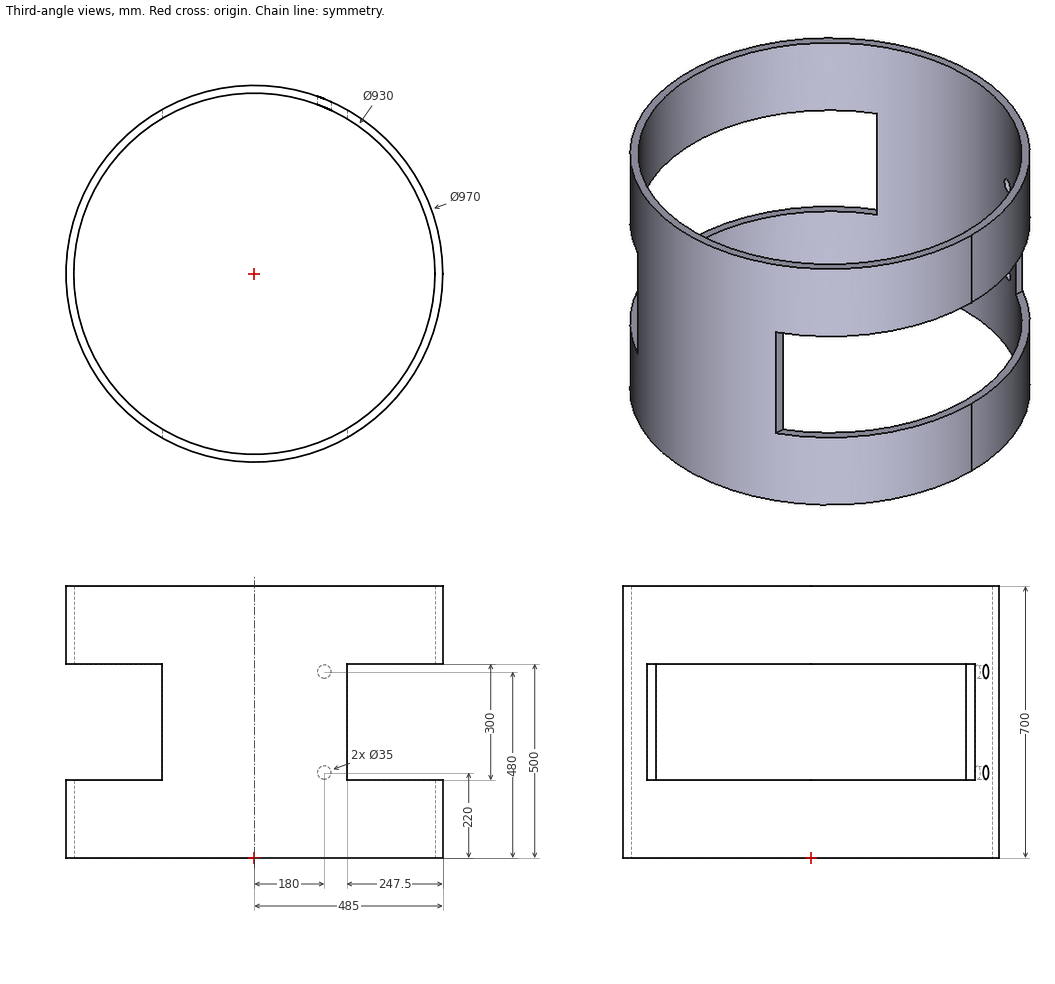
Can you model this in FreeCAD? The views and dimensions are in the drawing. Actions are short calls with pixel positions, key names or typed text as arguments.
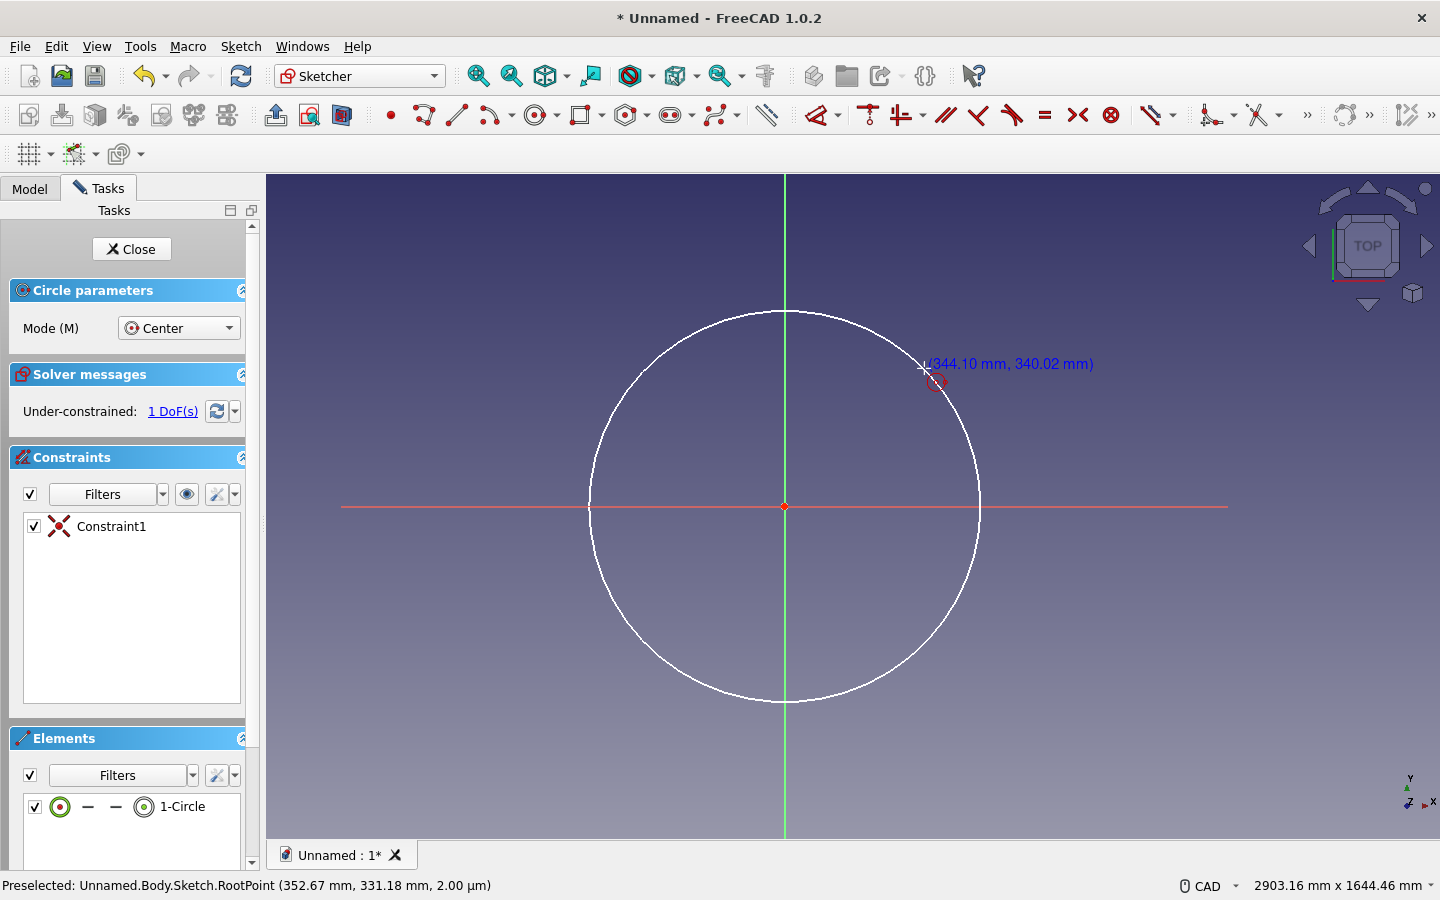
click(785, 506)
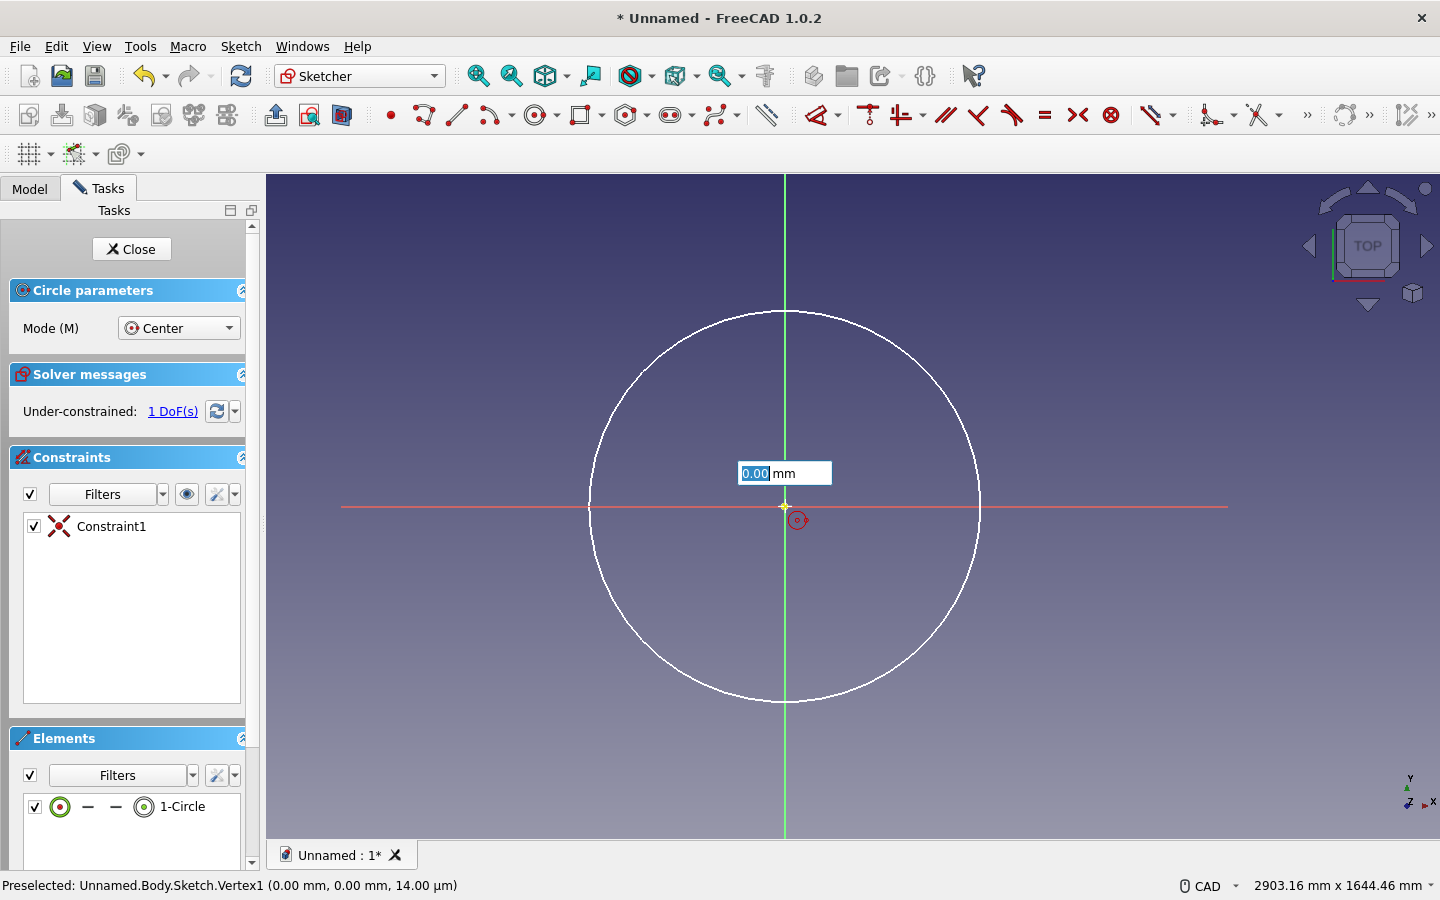
scroll(918, 374, up, 4)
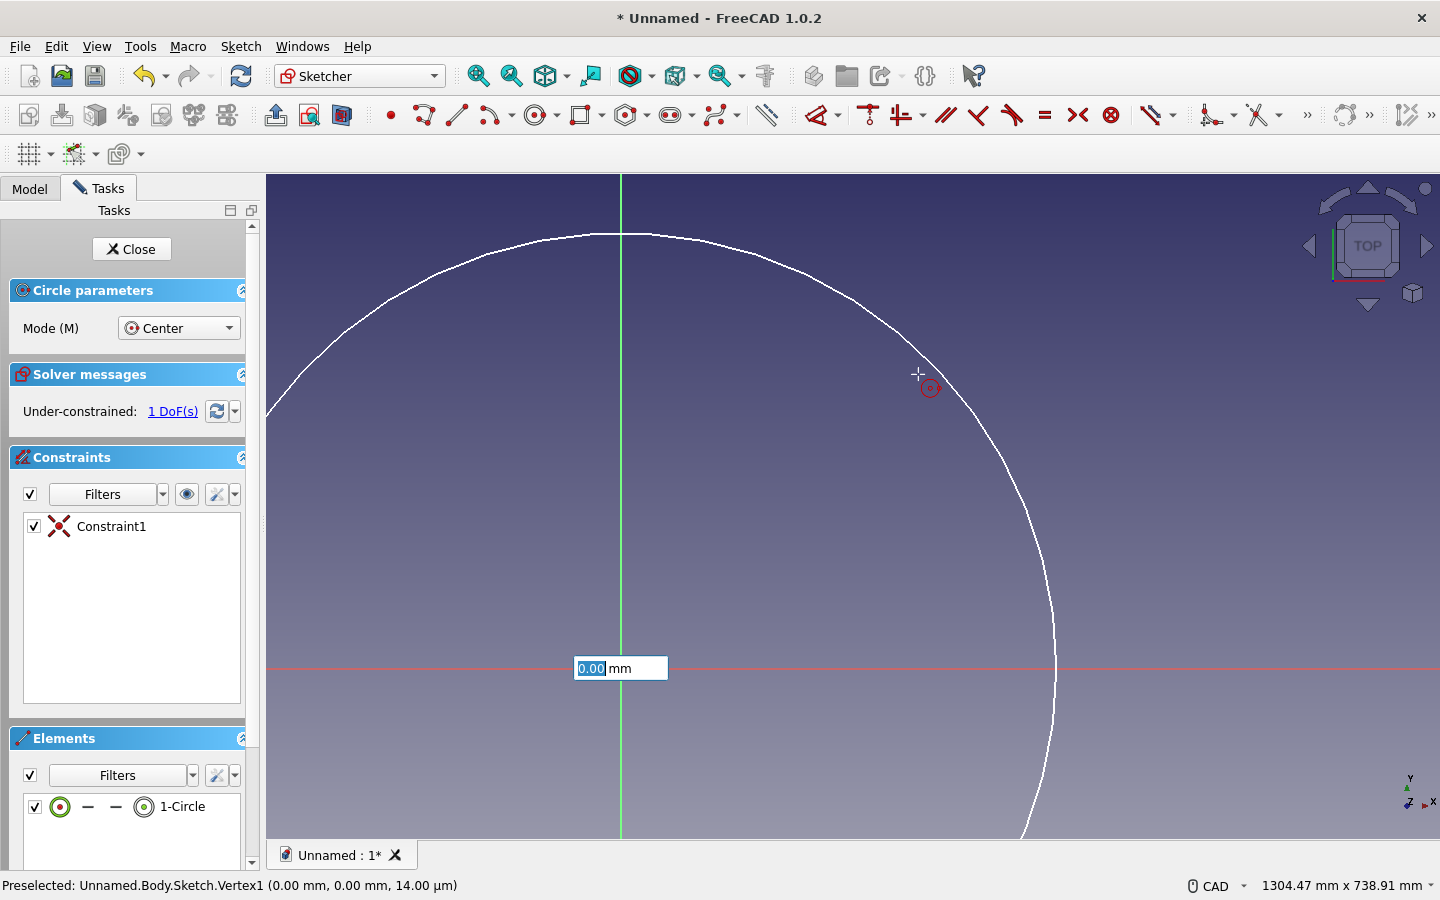
click(917, 373)
key(Escape)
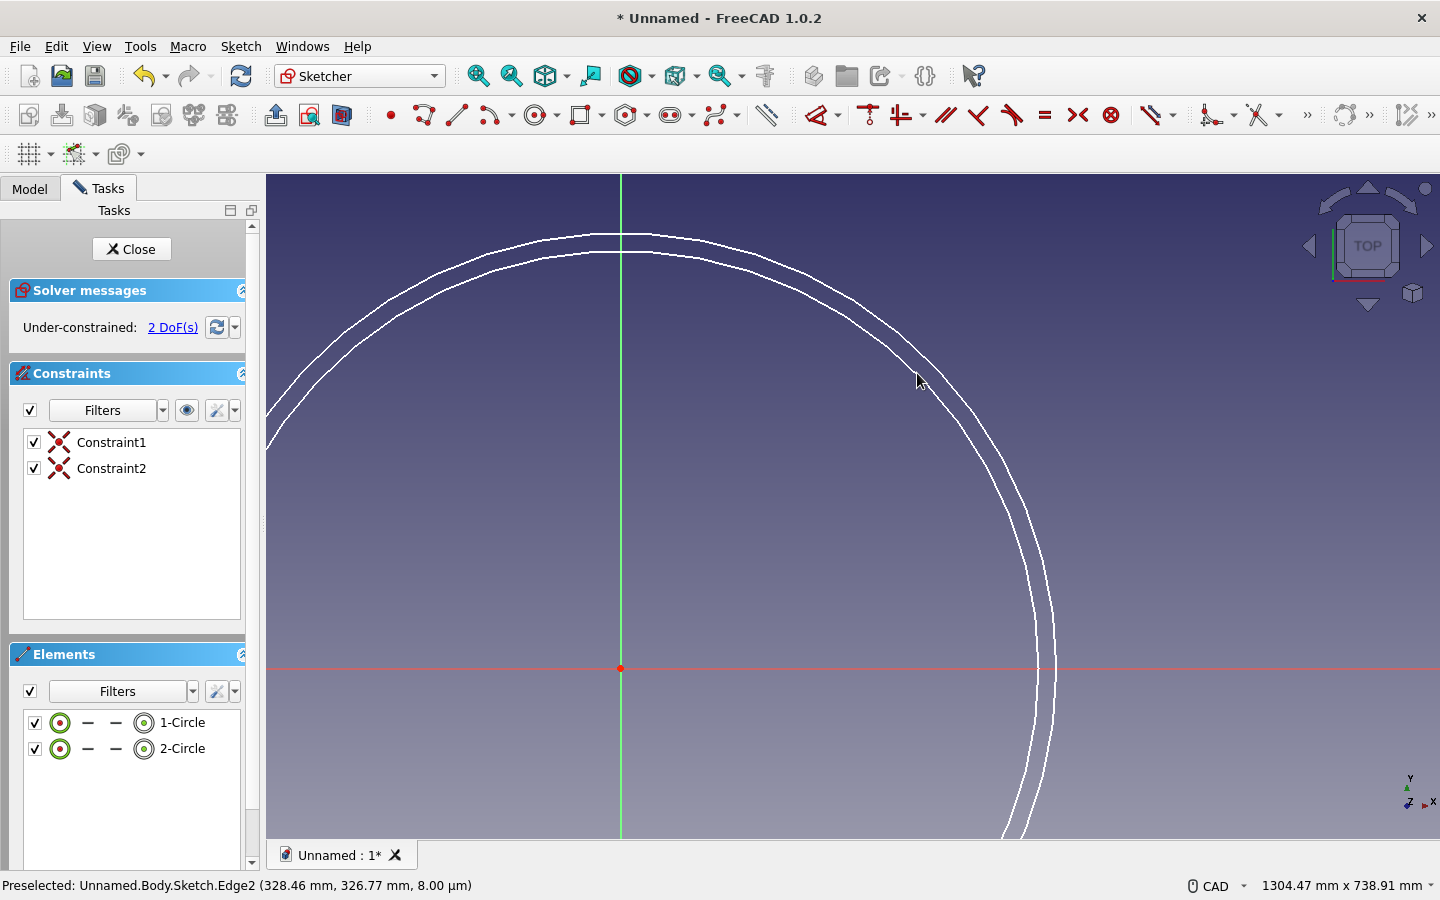
key(d)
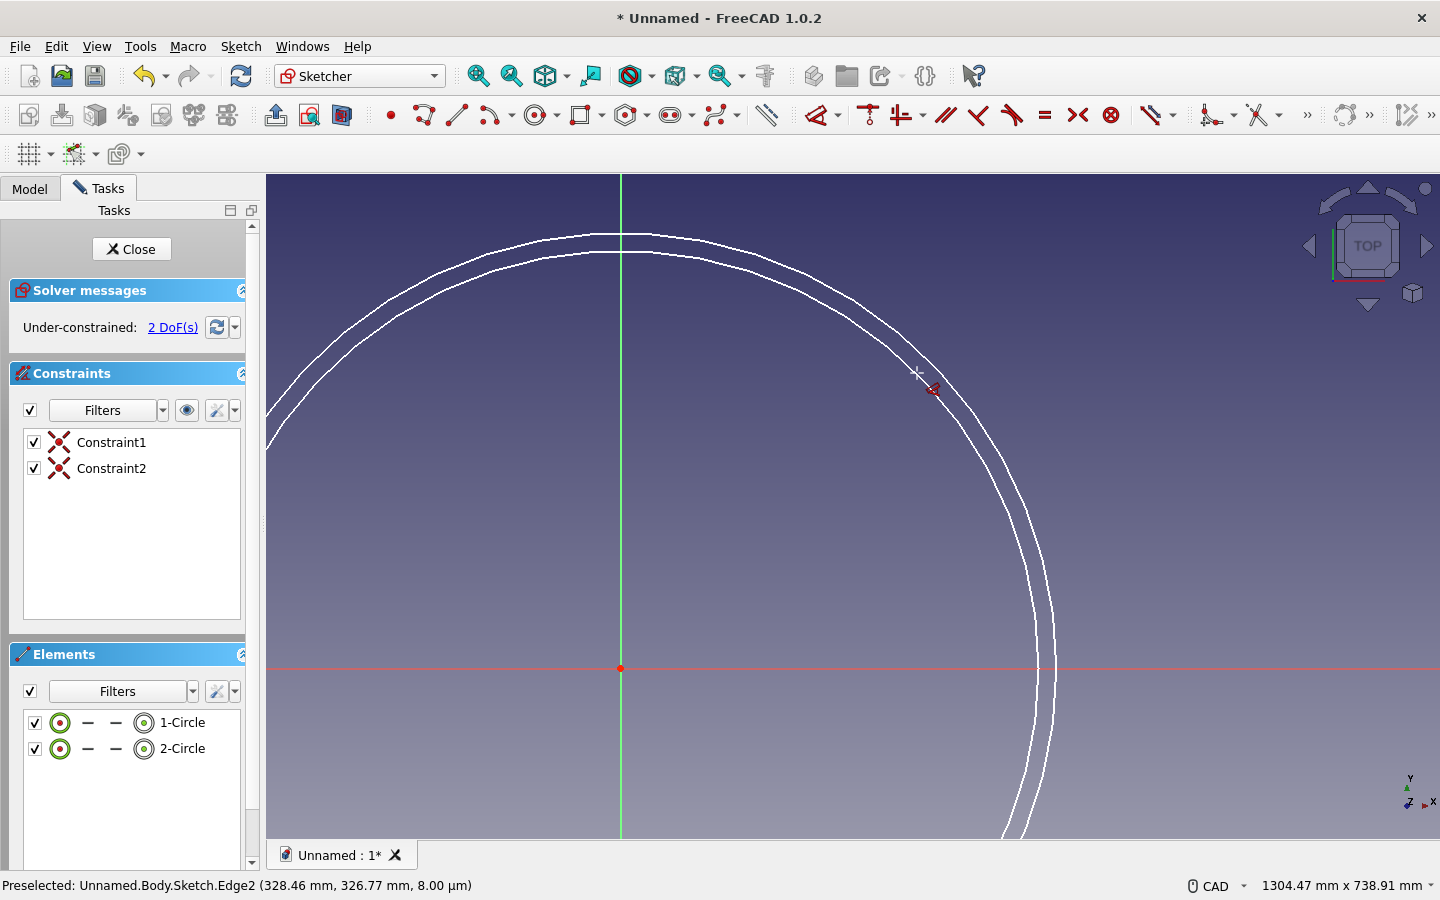
click(928, 360)
click(951, 337)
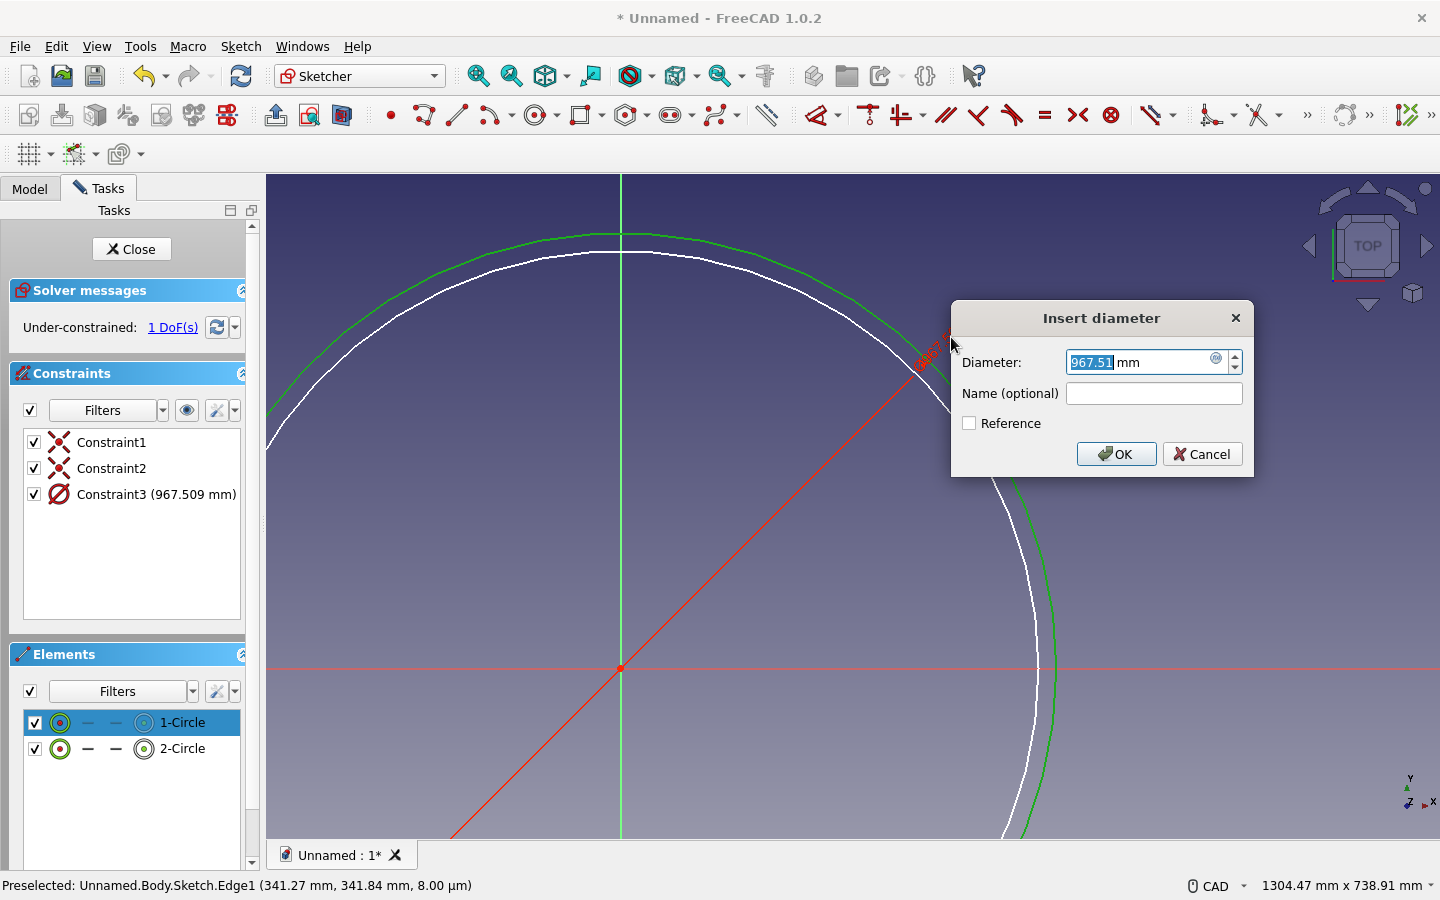
text(970)
key(Return)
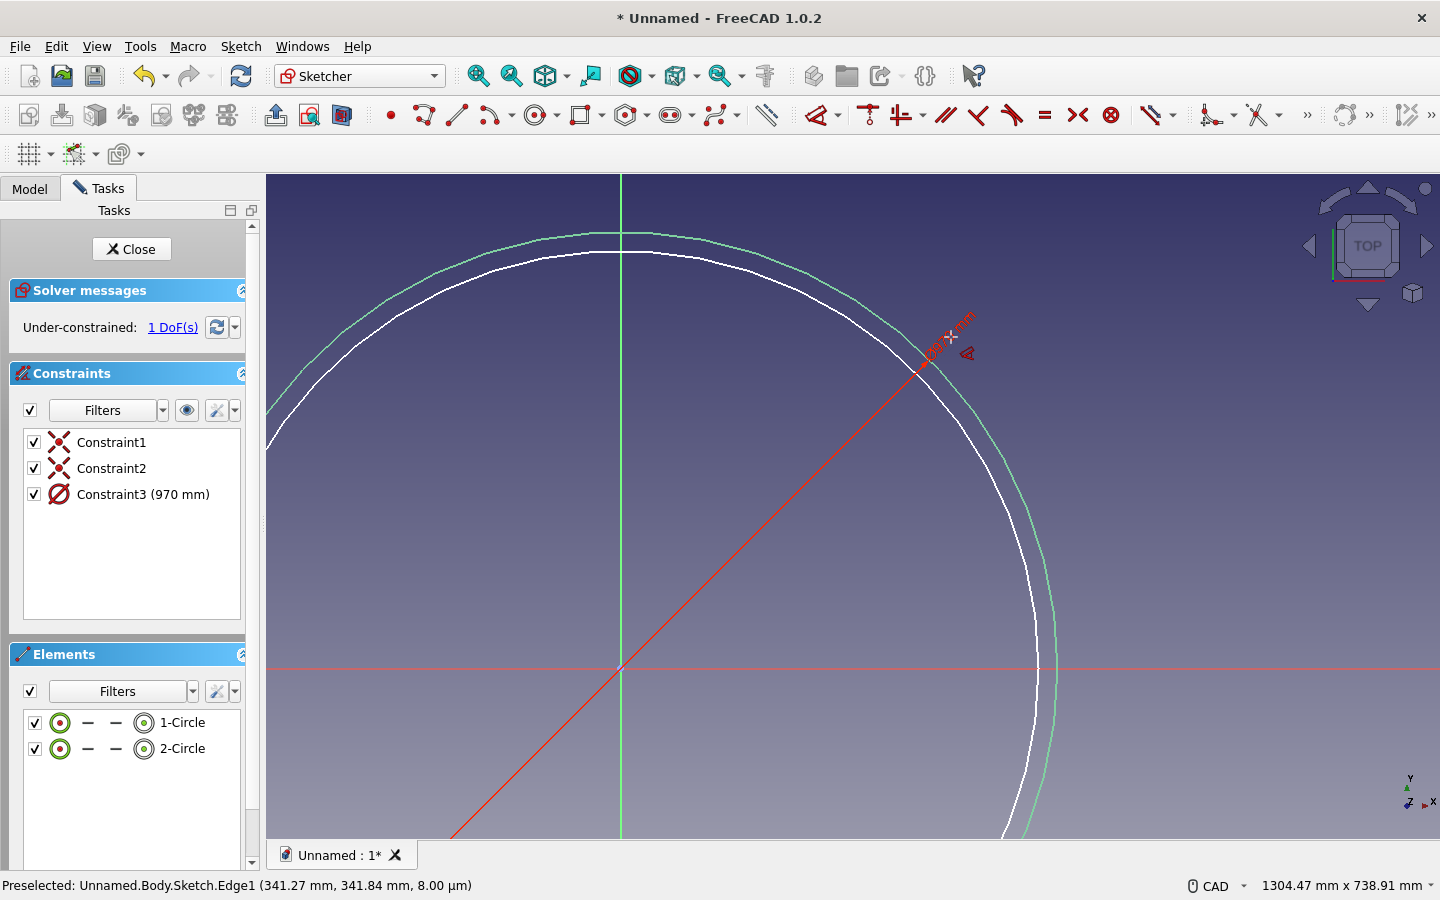
click(915, 372)
click(1052, 540)